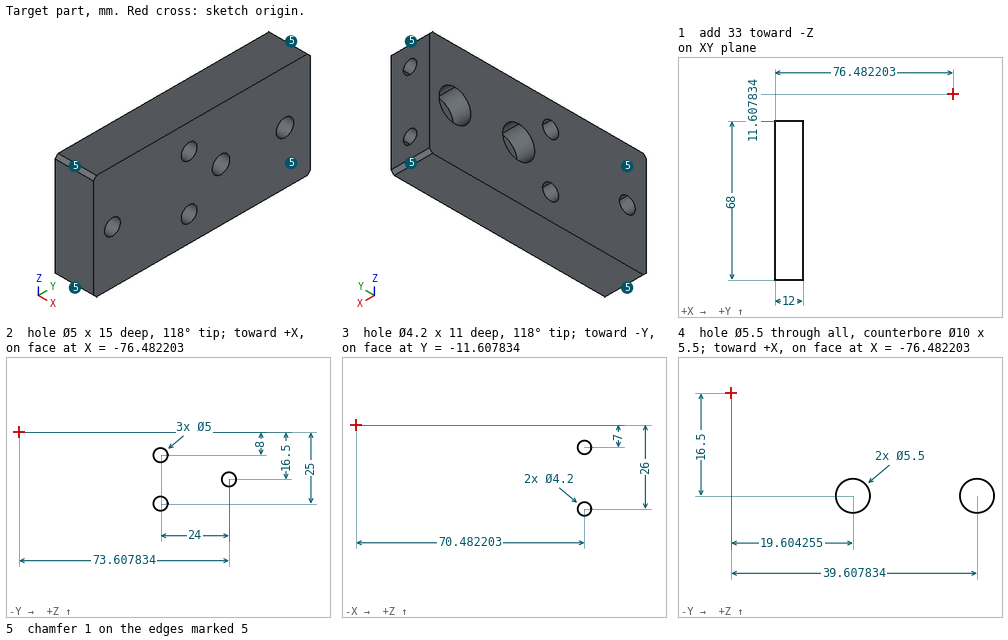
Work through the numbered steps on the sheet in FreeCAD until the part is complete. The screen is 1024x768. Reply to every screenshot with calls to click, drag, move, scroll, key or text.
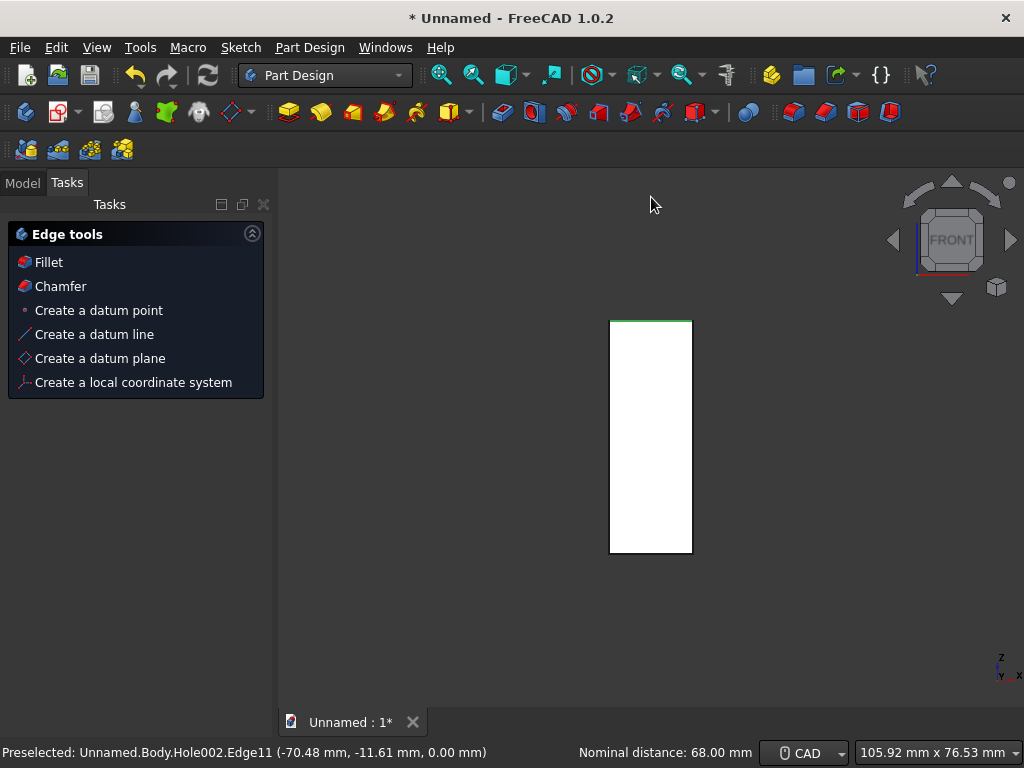
click(442, 76)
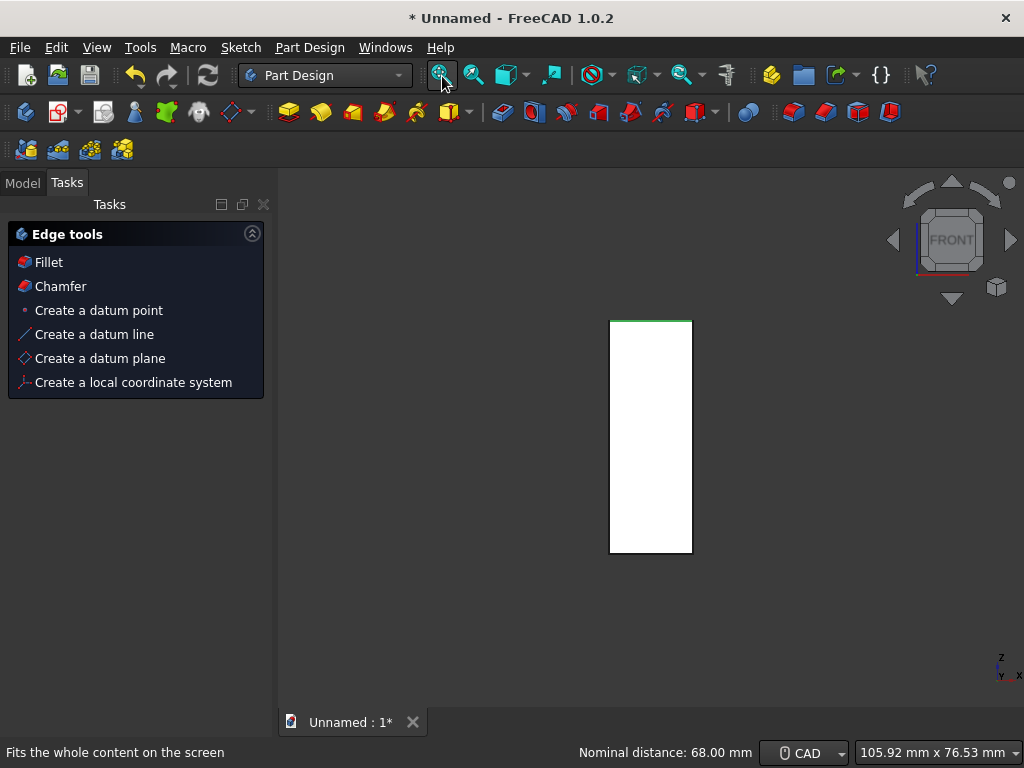
click(651, 553, ctrl)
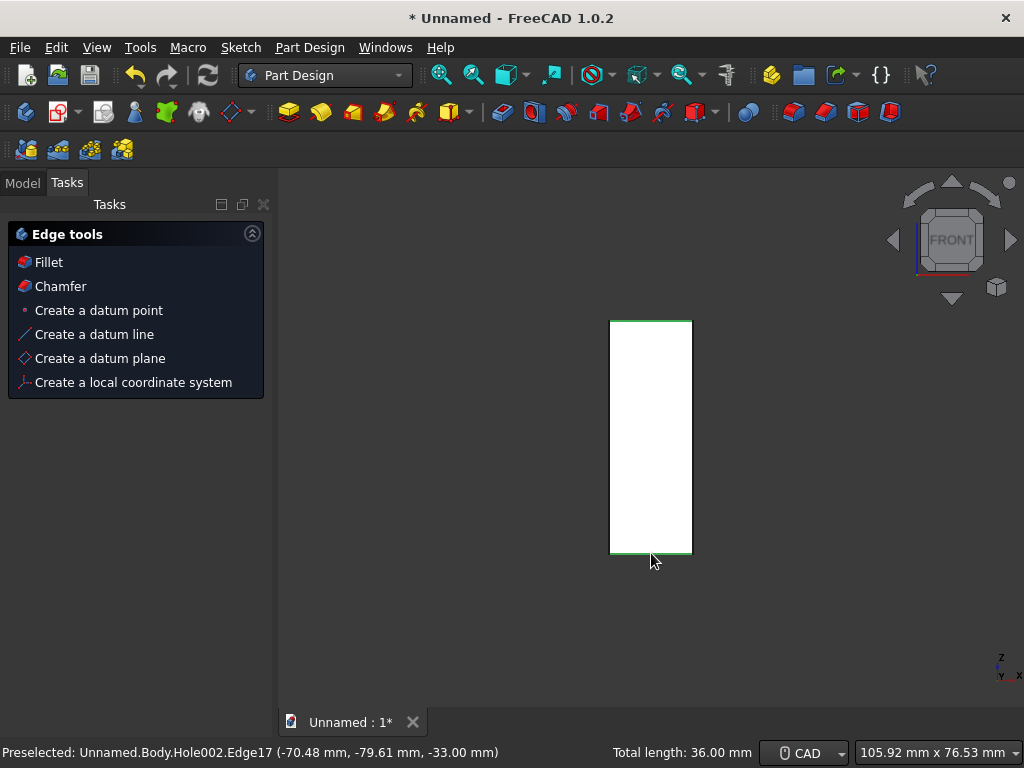
key(3)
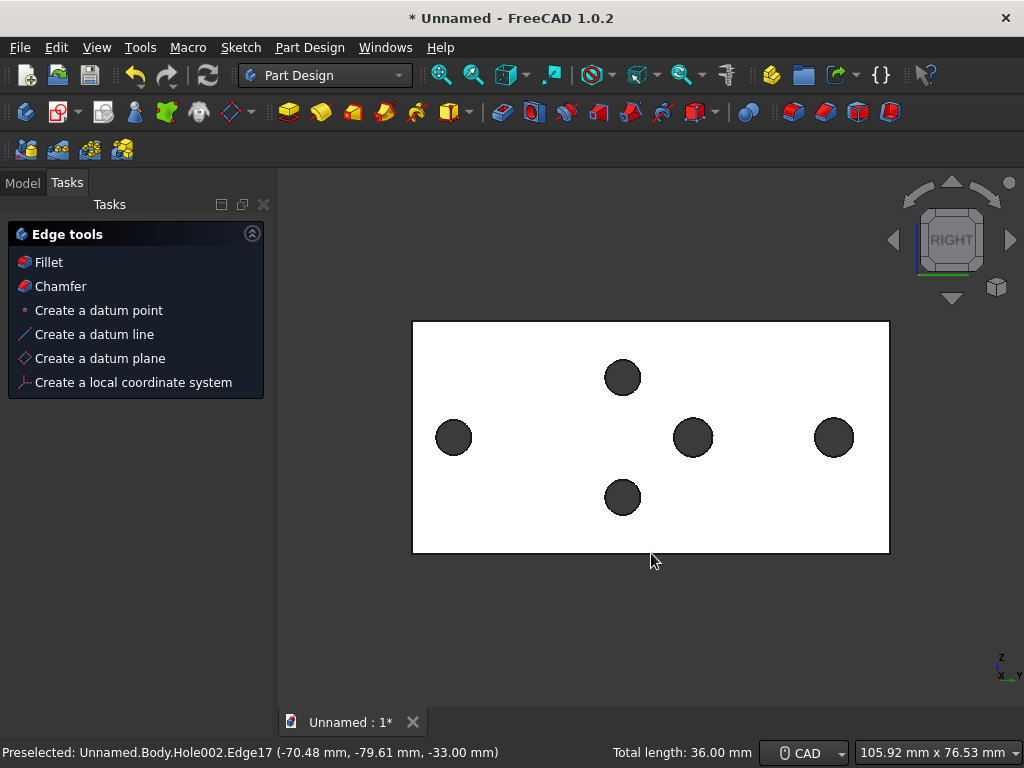
key(5)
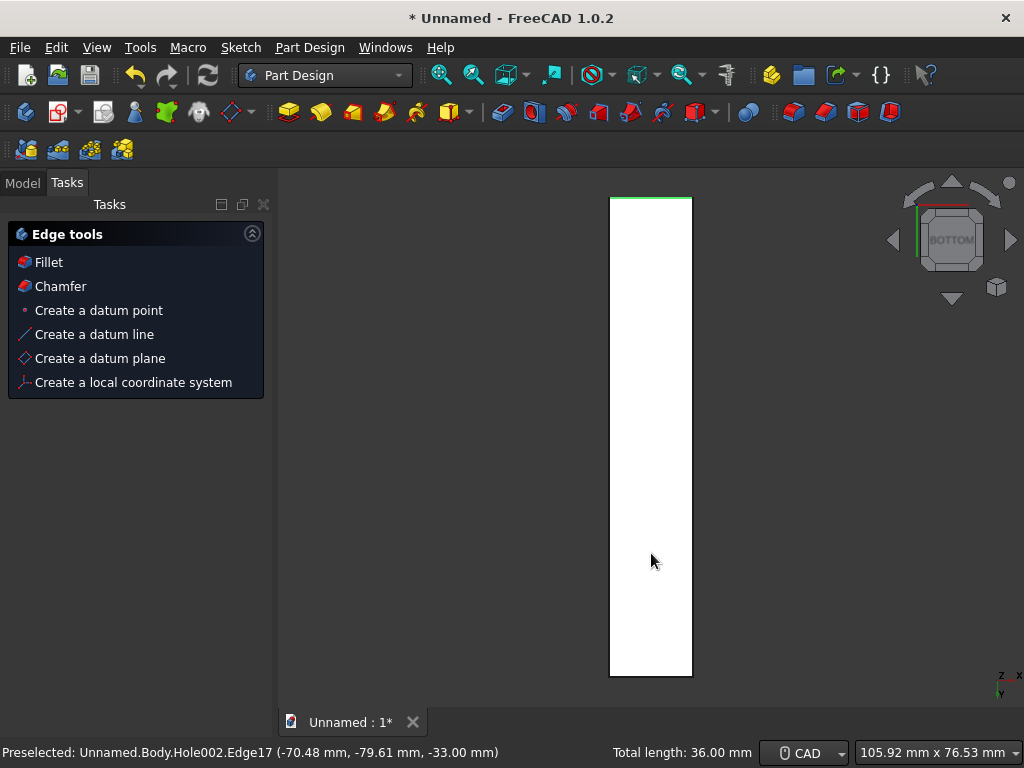
click(651, 676, ctrl)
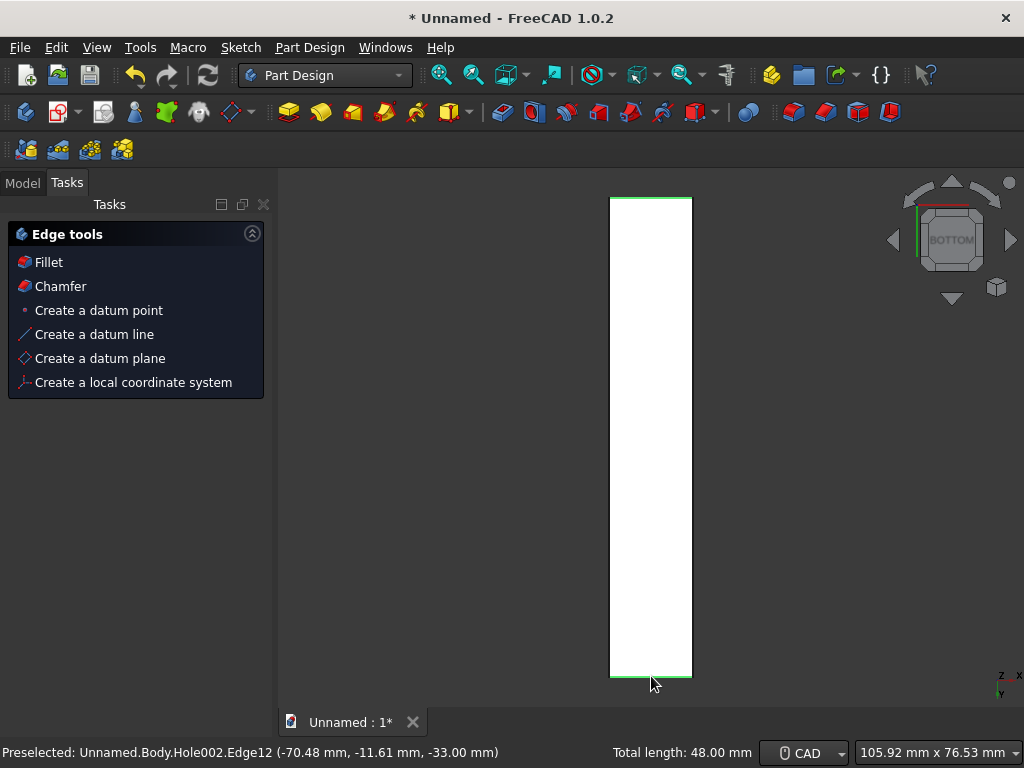
click(826, 112)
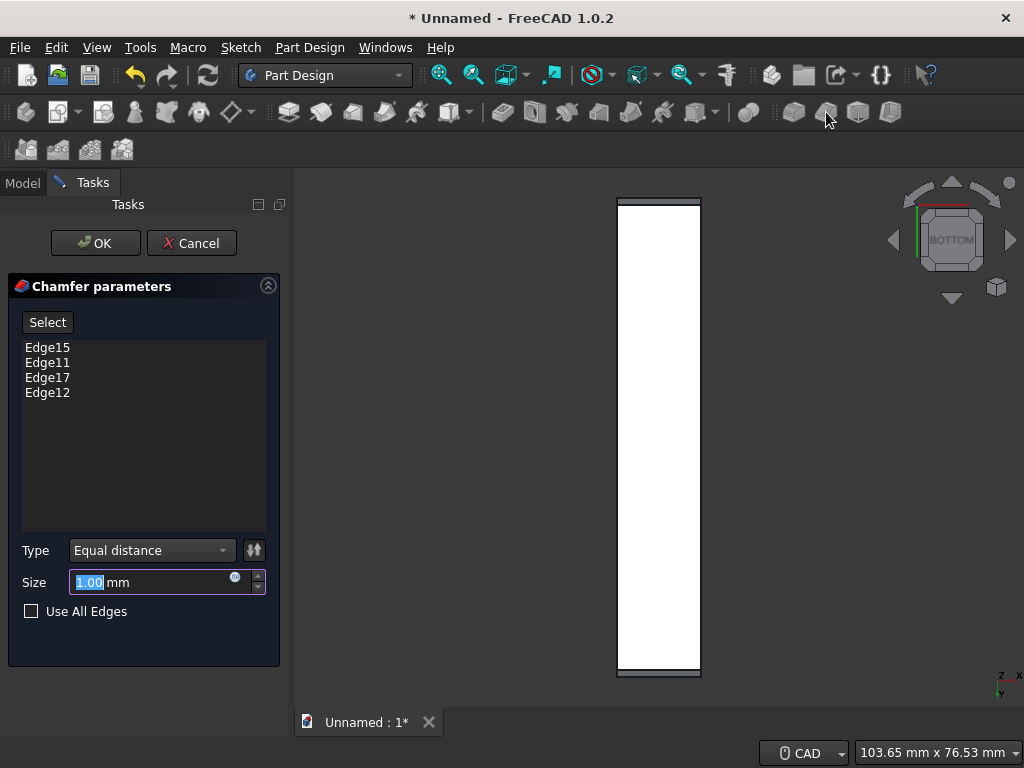
text(1)
key(Tab)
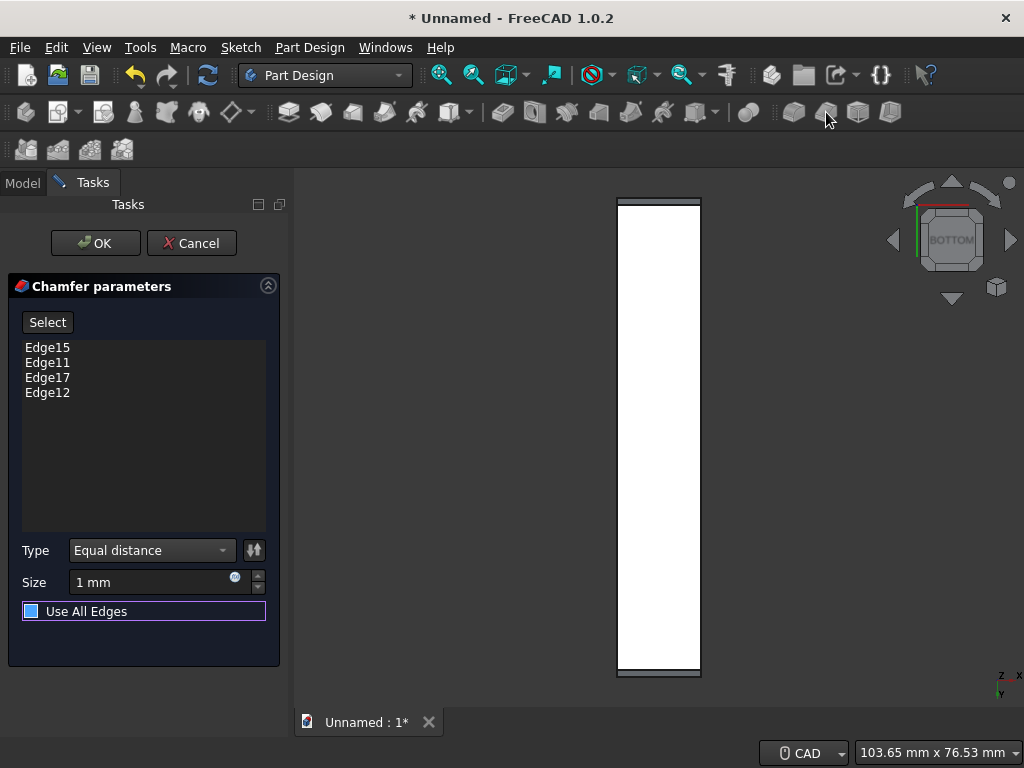
click(96, 243)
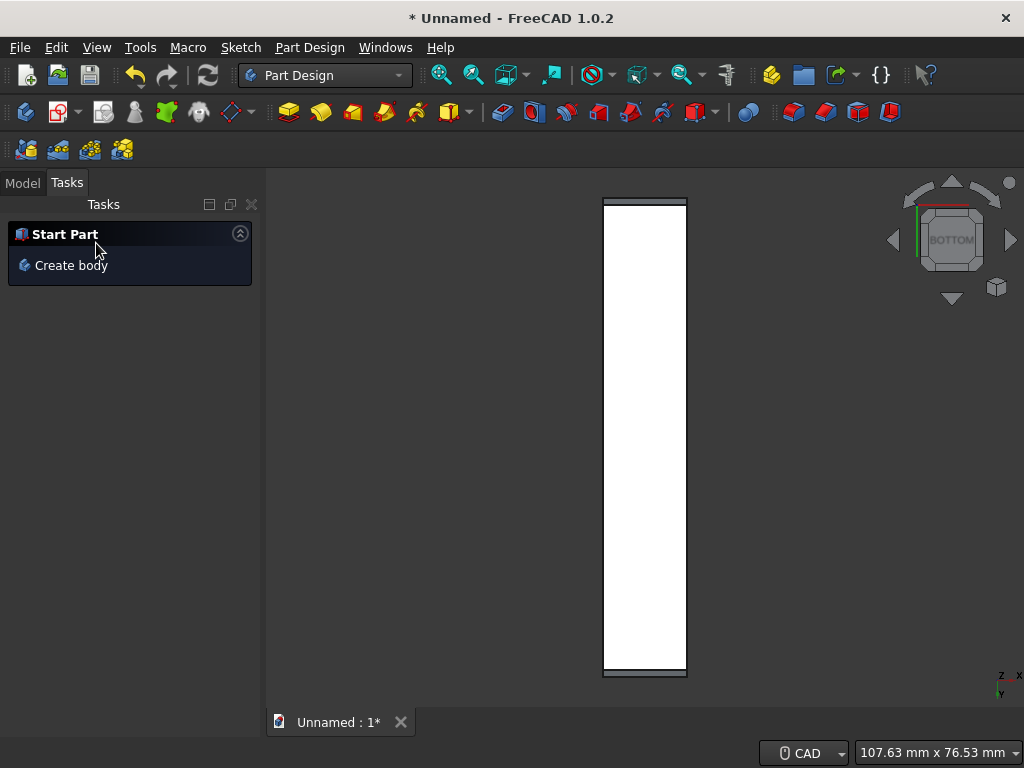
key(0)